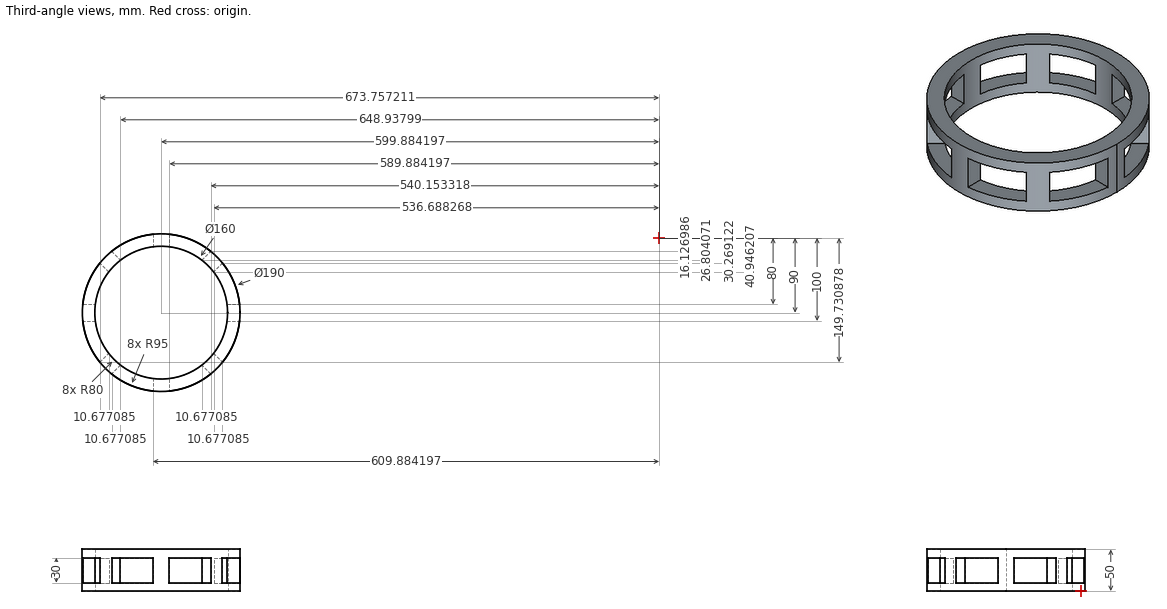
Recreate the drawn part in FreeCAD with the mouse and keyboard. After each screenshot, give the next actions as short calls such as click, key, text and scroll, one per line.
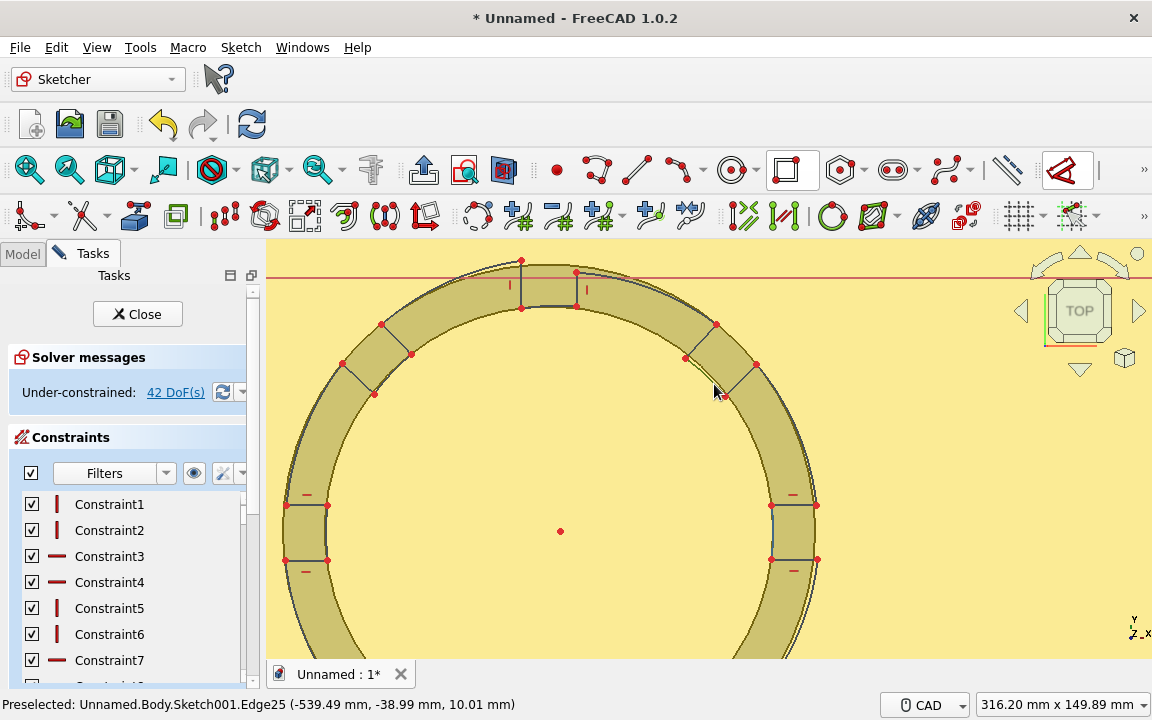
click(560, 306)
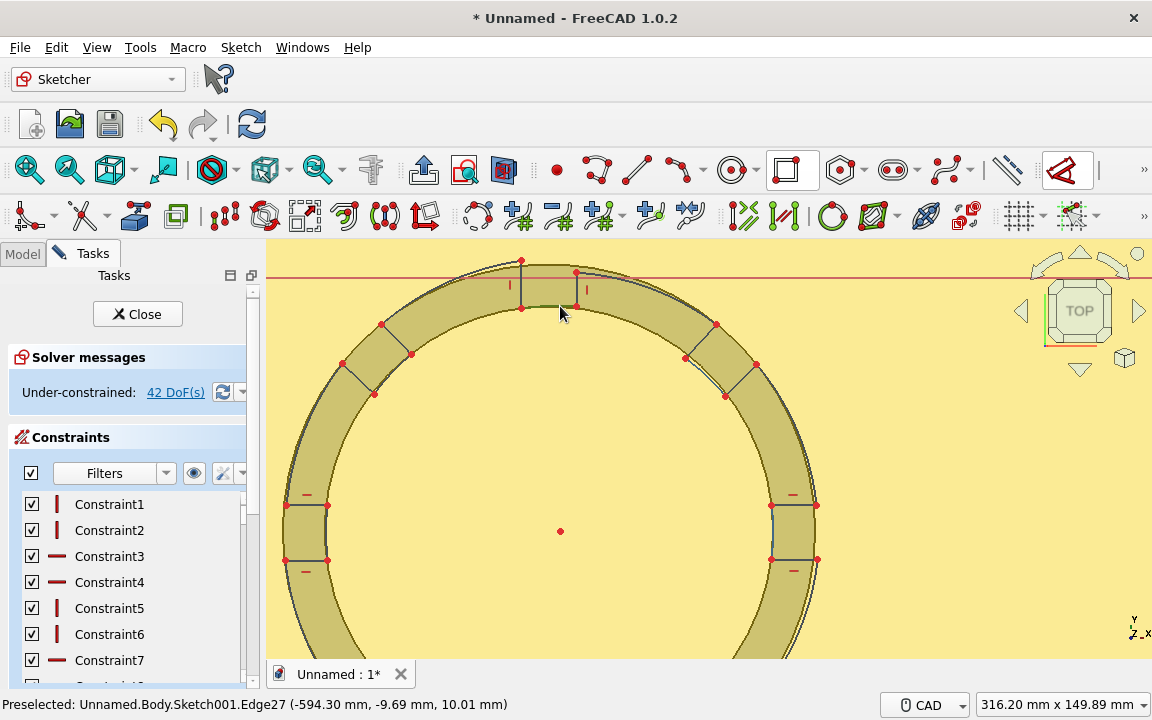
click(399, 365)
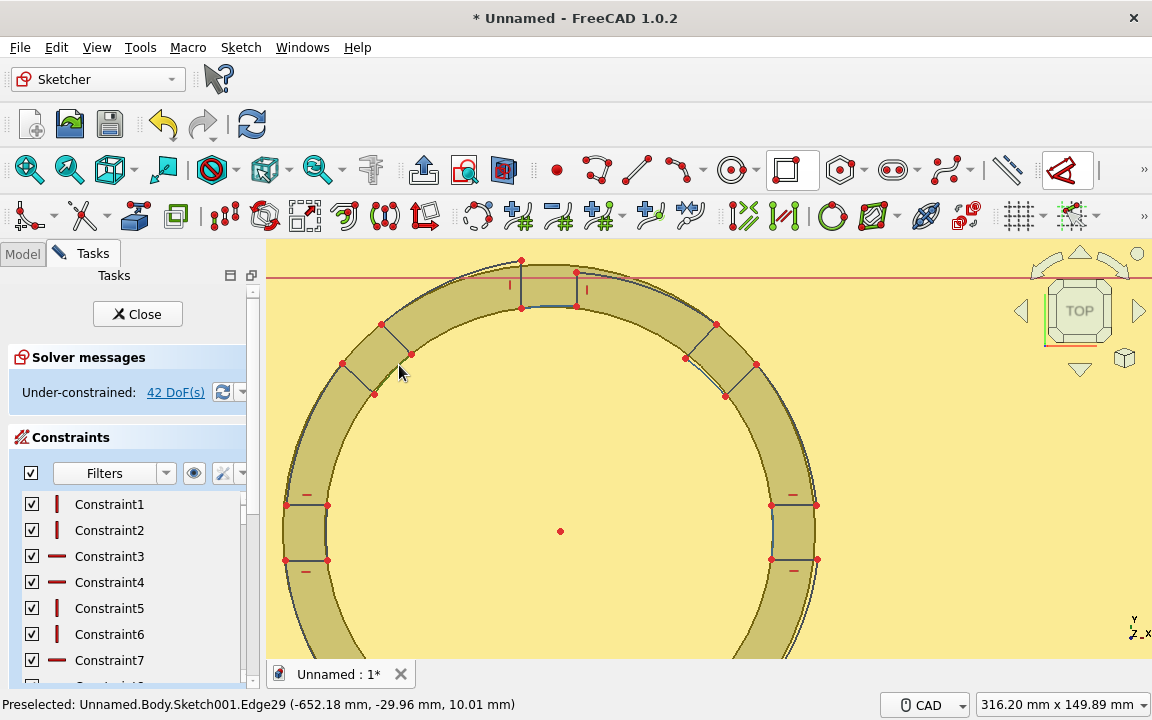
click(326, 522)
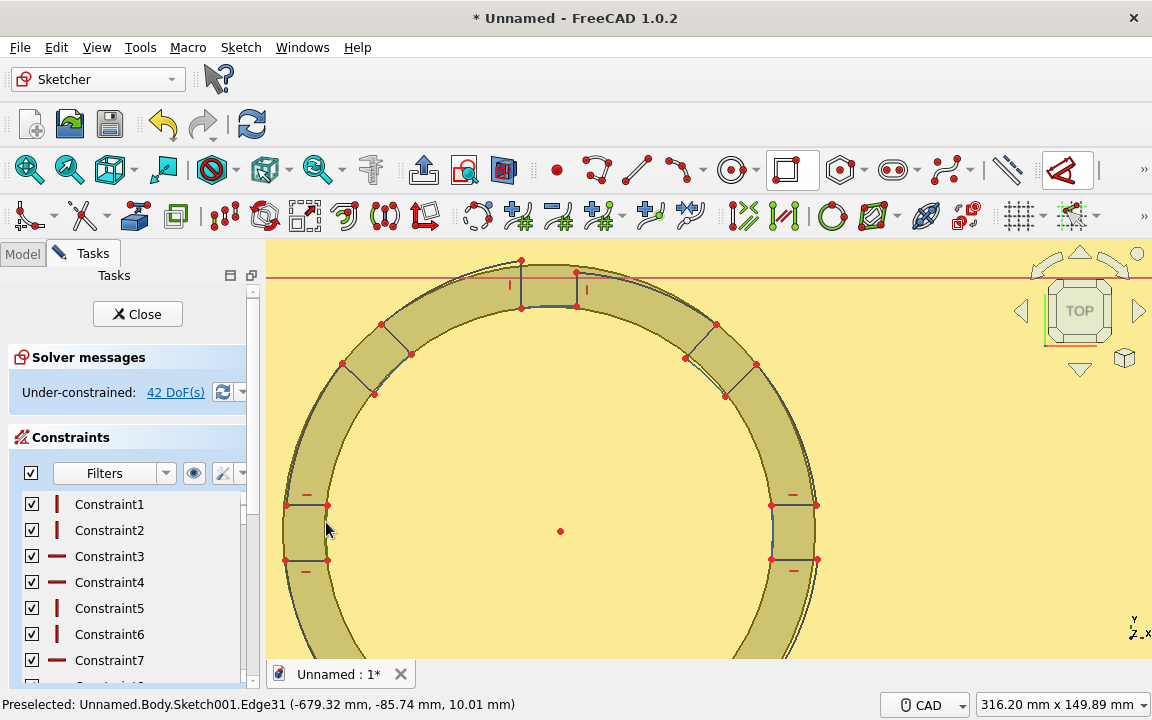
key(e)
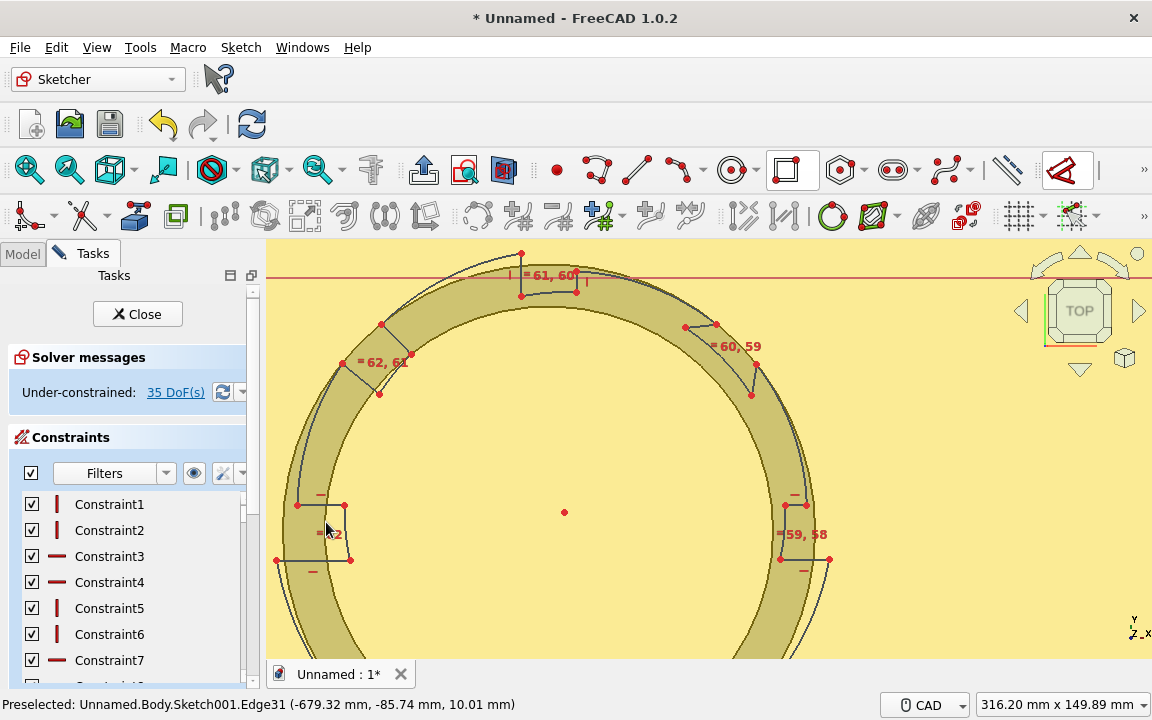
scroll(715, 382, down, 4)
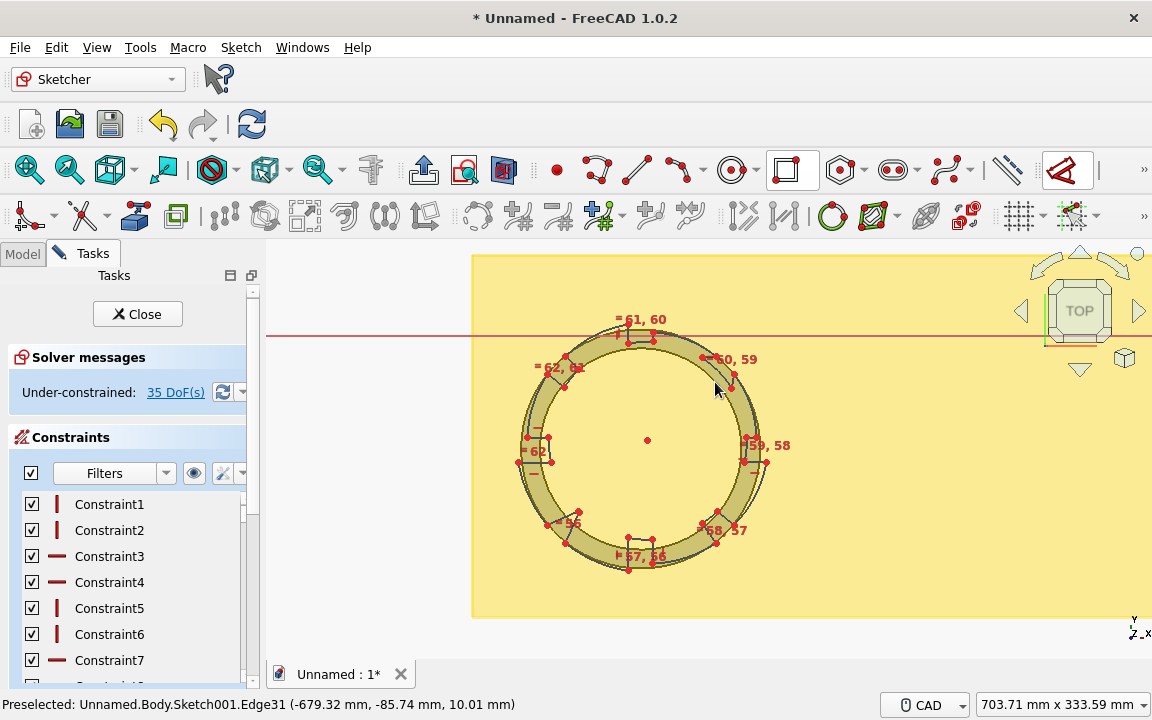
click(583, 555)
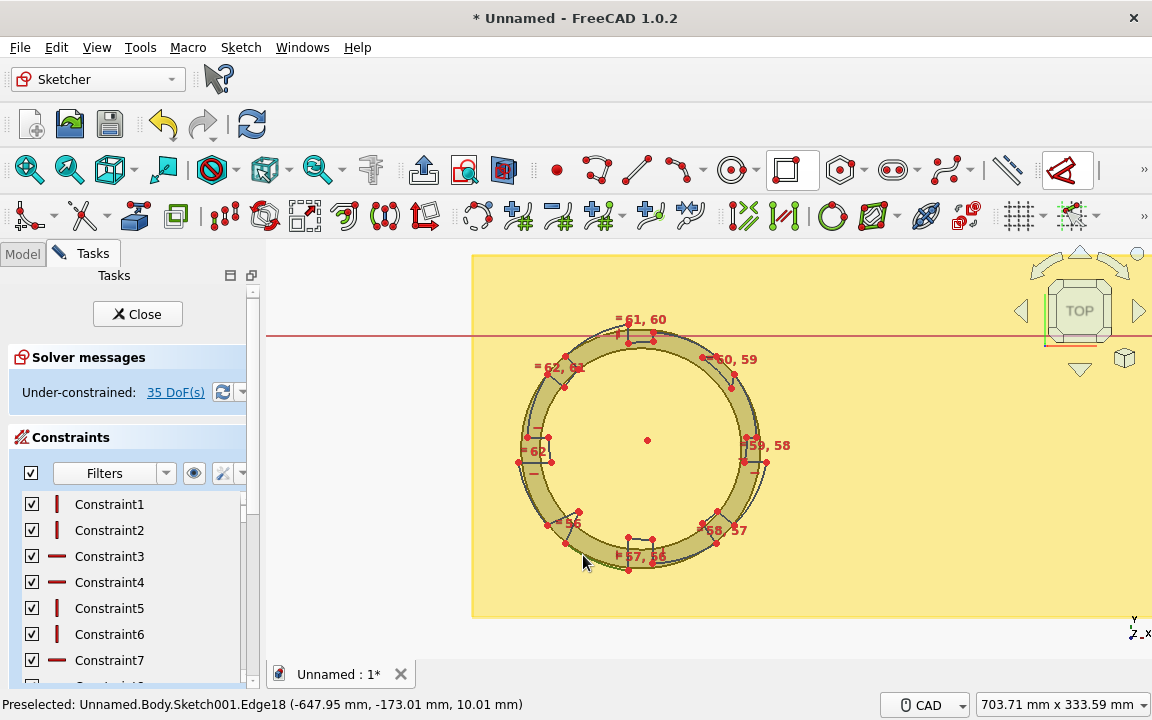
click(673, 561)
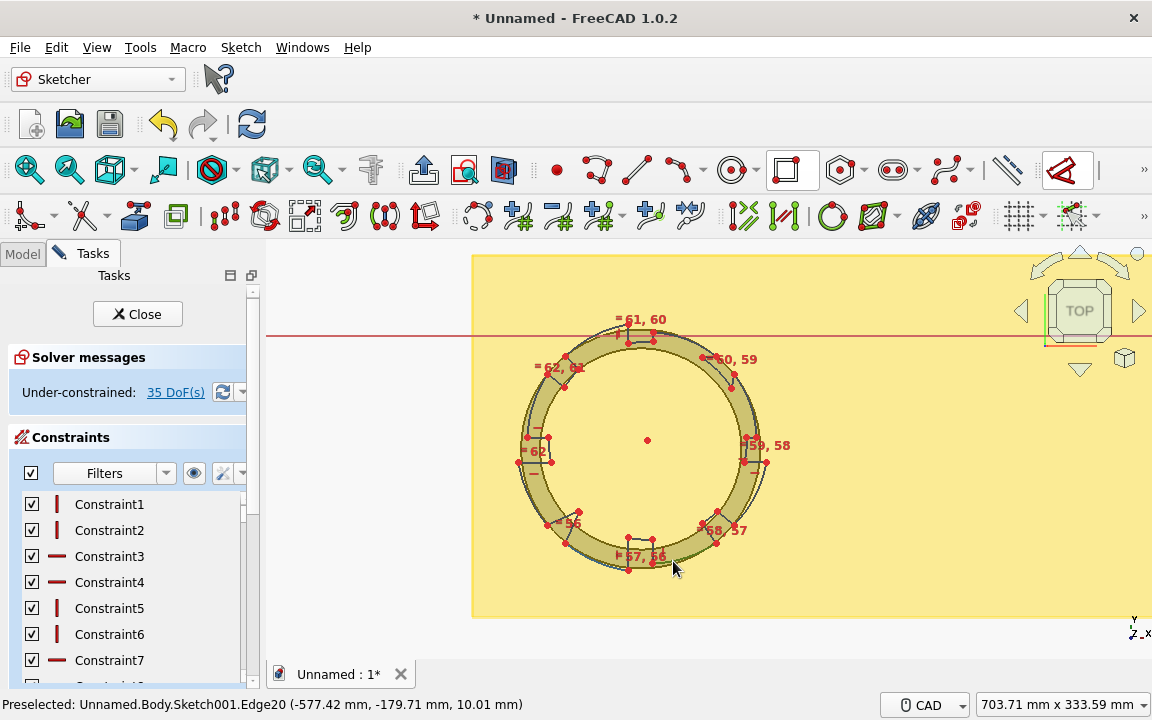
click(748, 508)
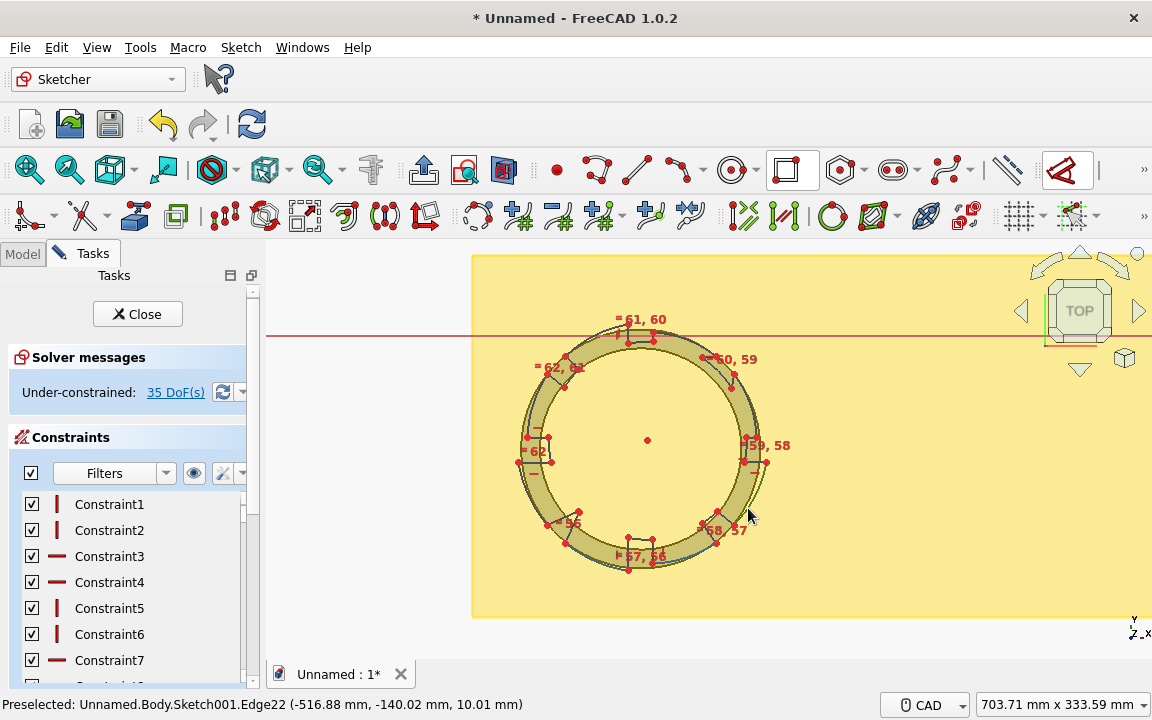
click(754, 417)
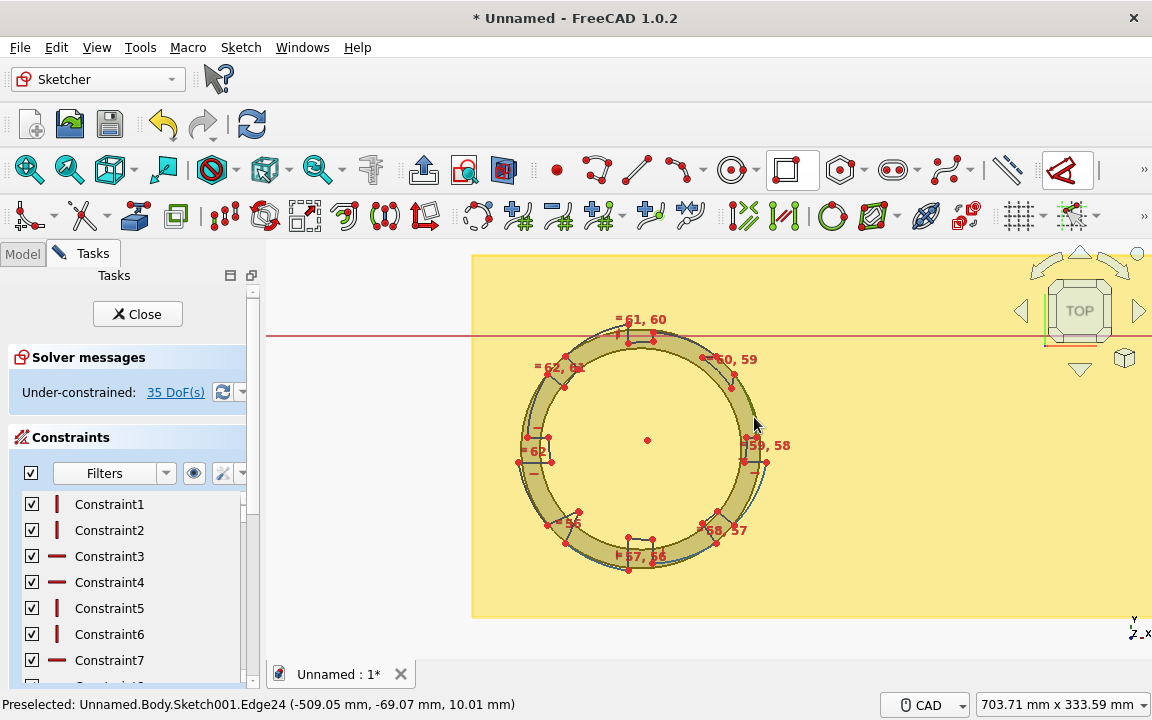
scroll(699, 345, up, 2)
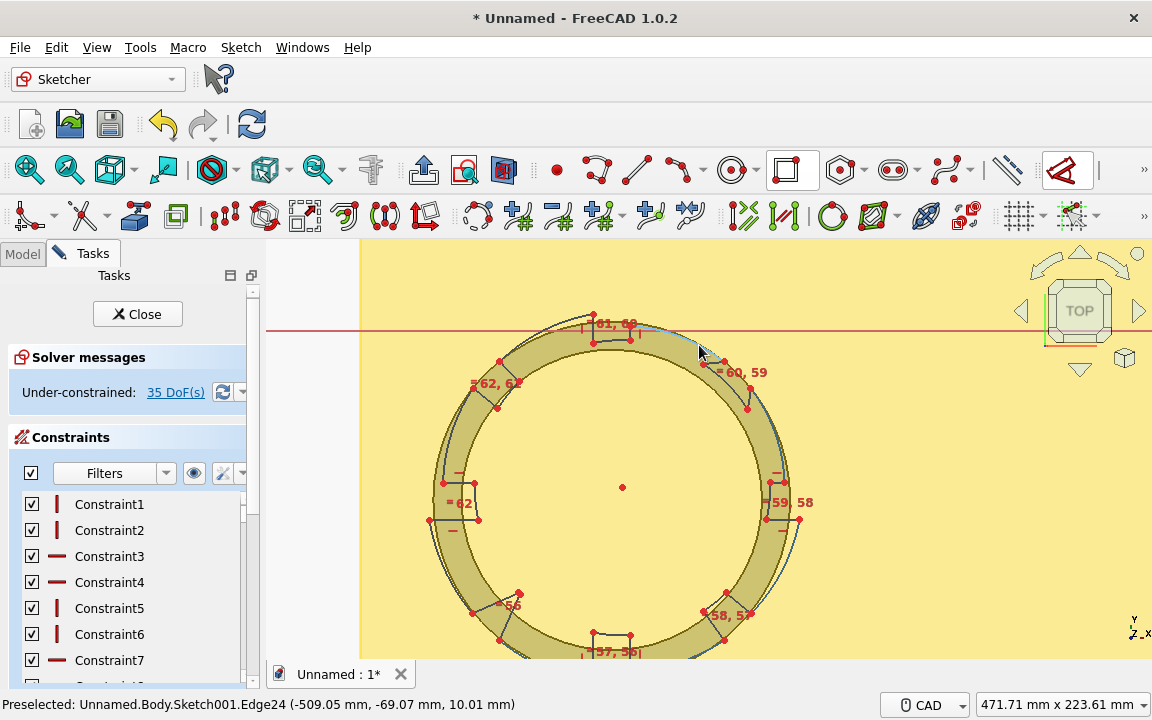
click(699, 345)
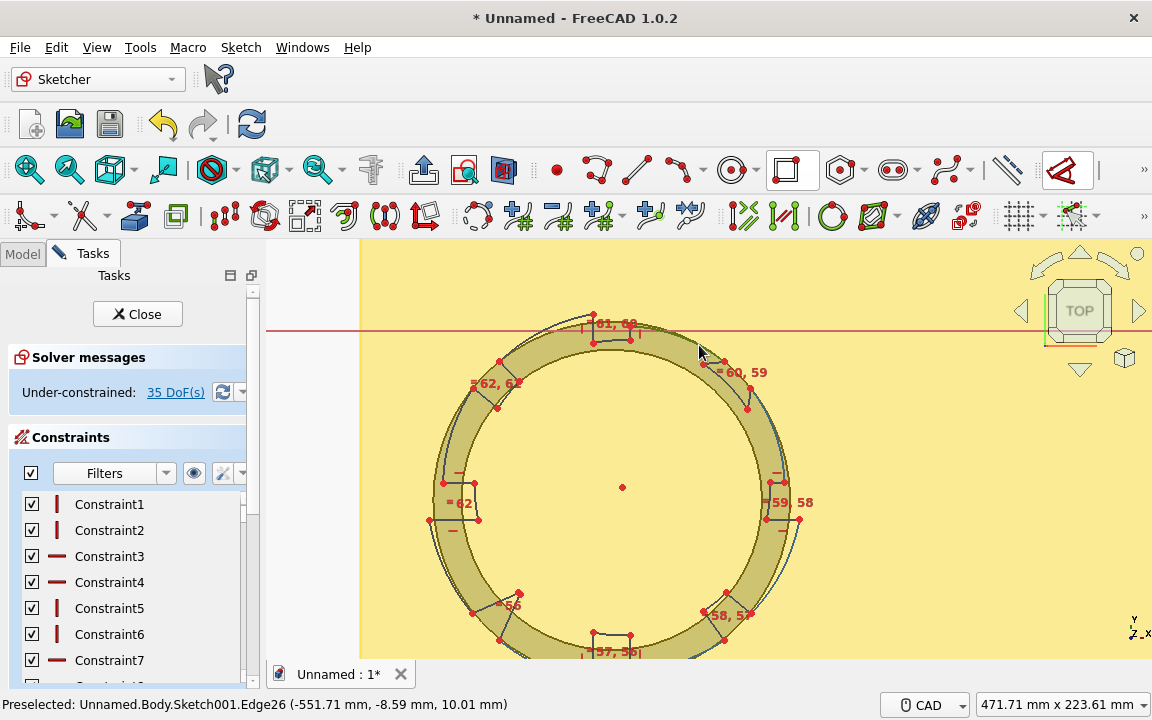
scroll(524, 342, up, 2)